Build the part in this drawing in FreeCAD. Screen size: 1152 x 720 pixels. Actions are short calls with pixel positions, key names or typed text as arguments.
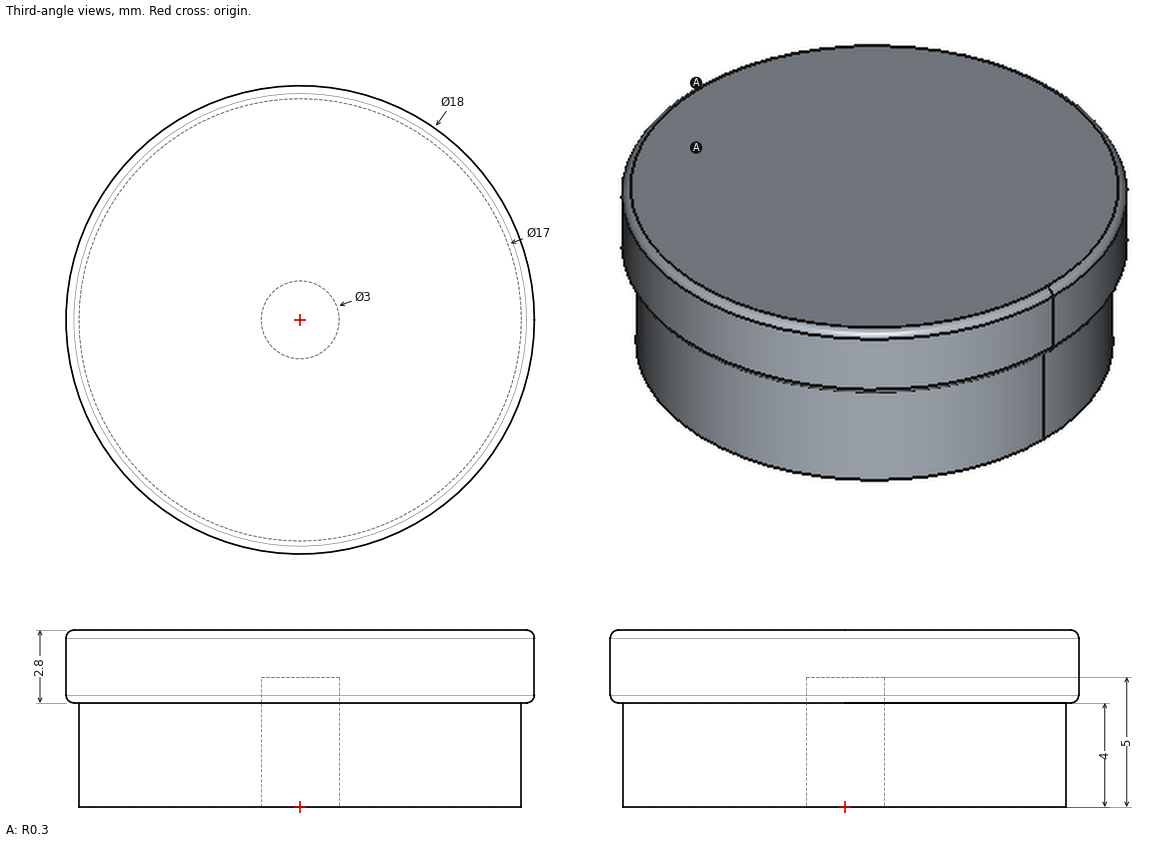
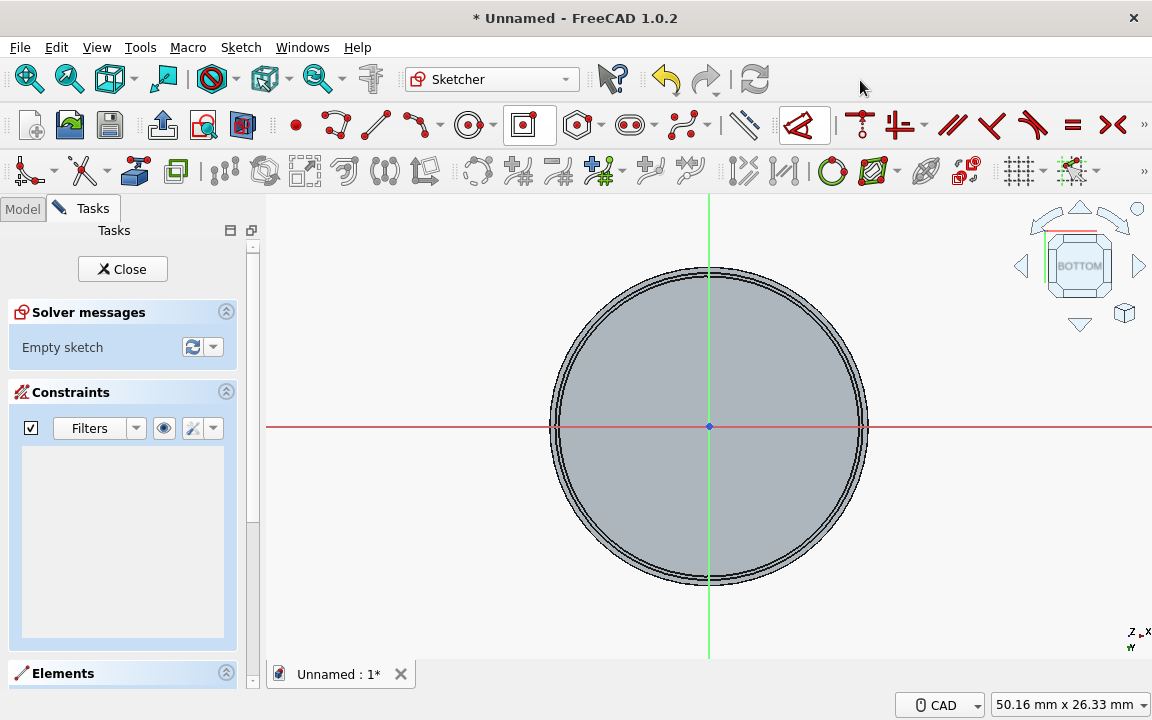
scroll(726, 426, up, 8)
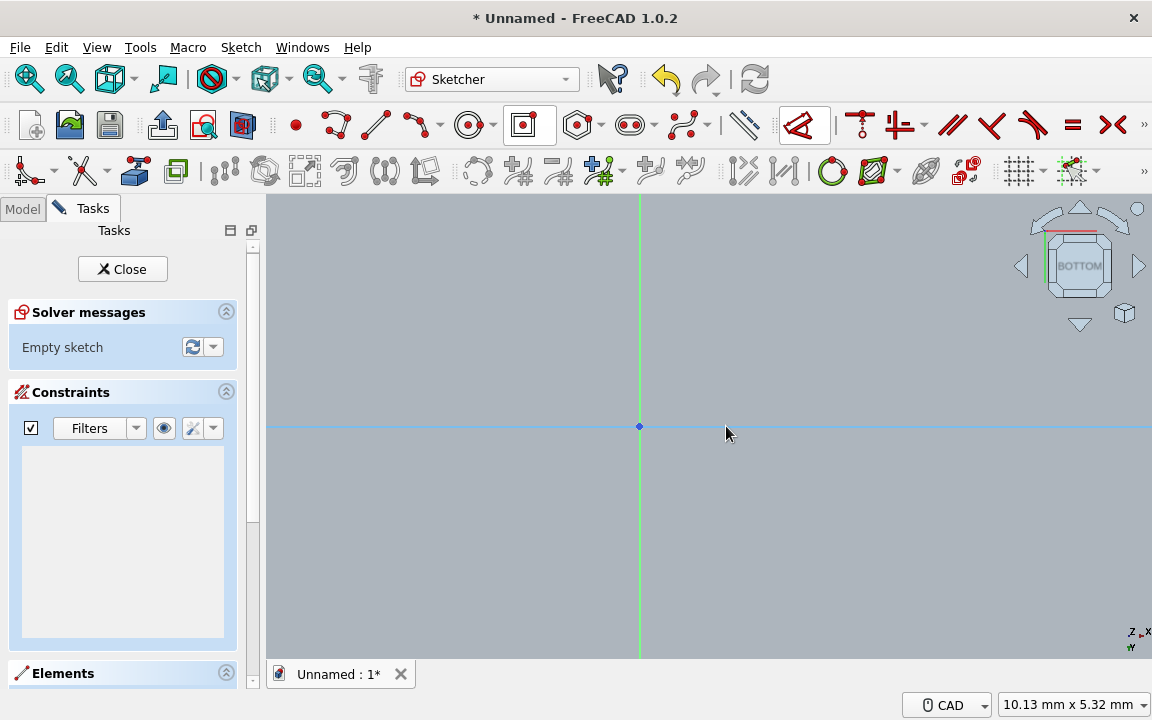
key(g)
key(c)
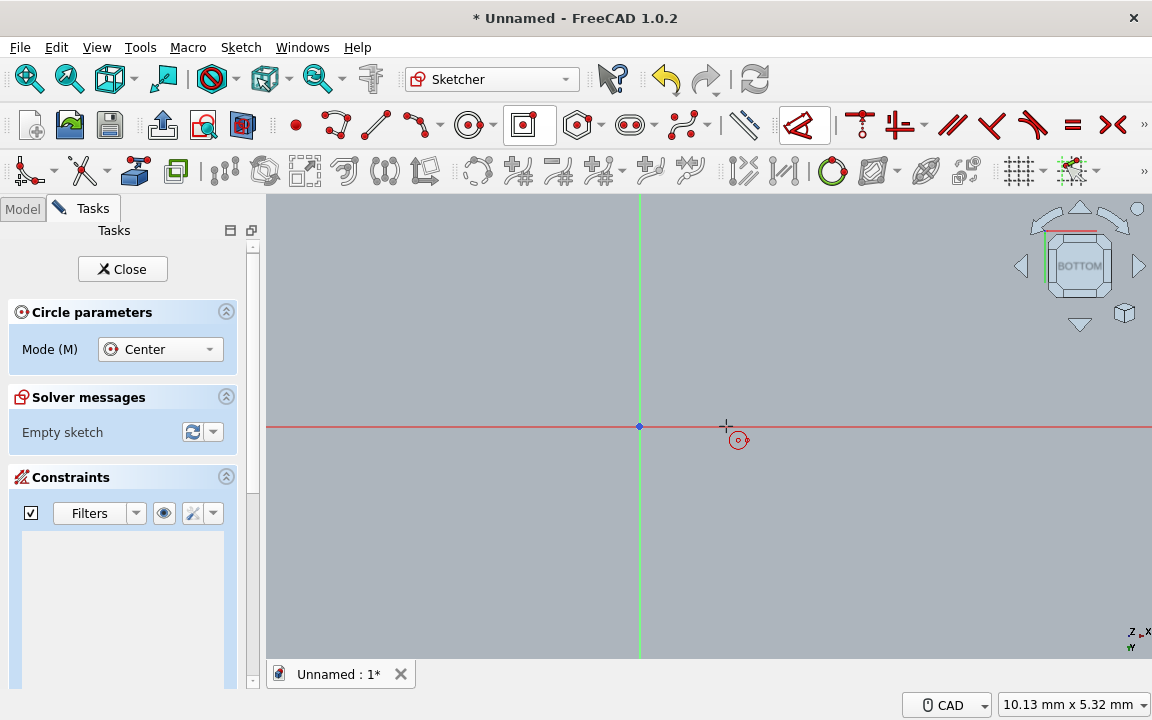
click(640, 426)
move(733, 334)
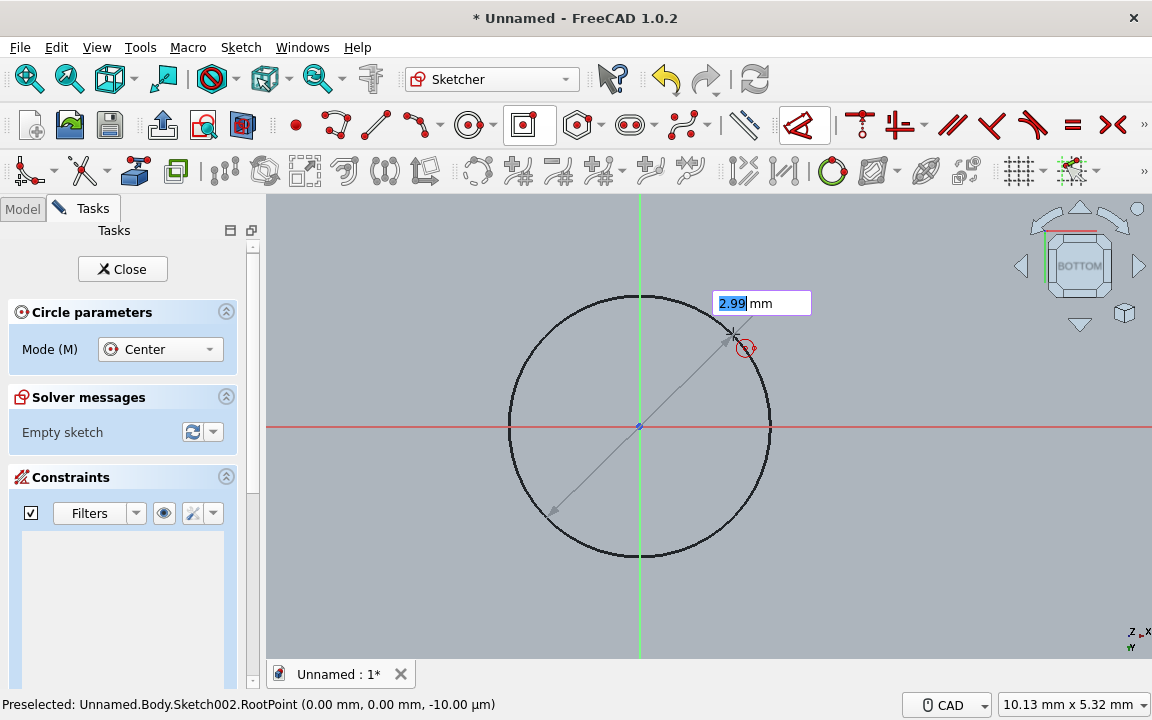
text(3)
key(Return)
key(Escape)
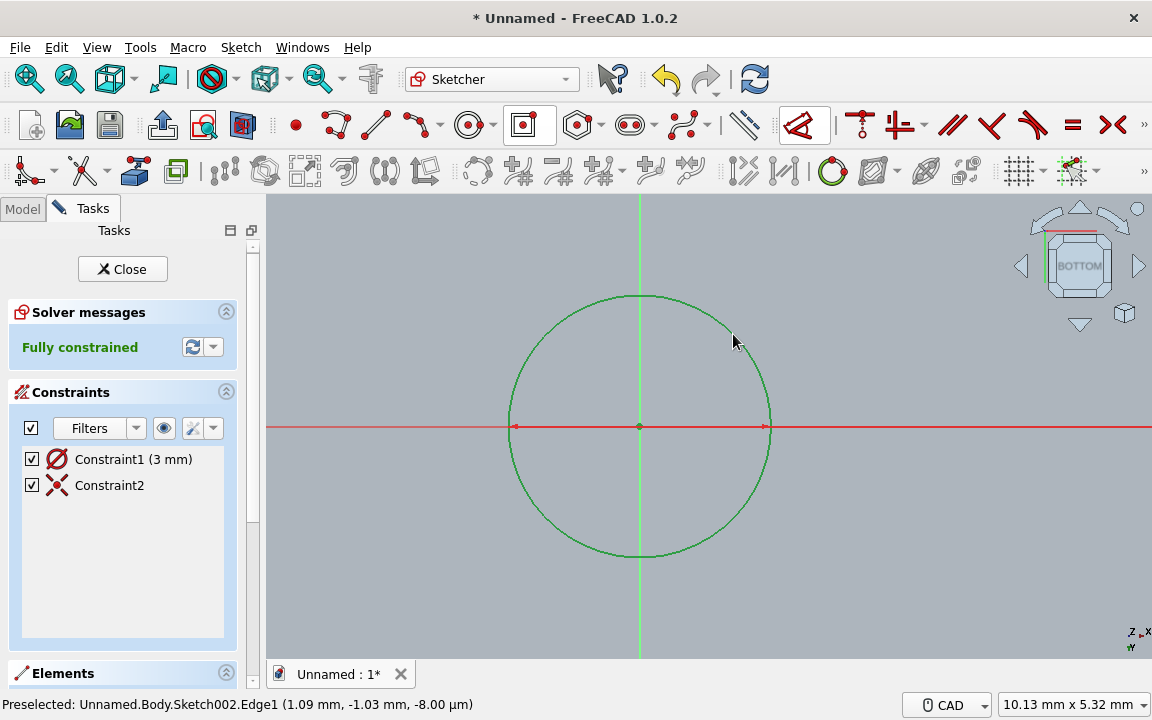
click(123, 269)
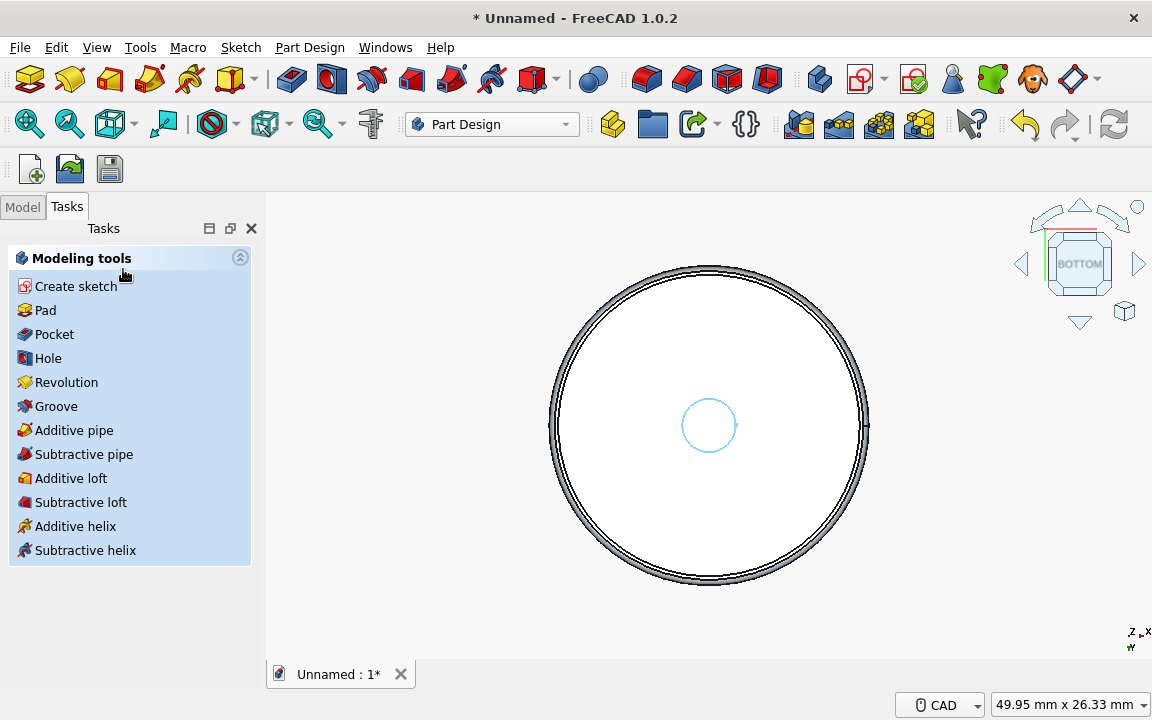
click(292, 80)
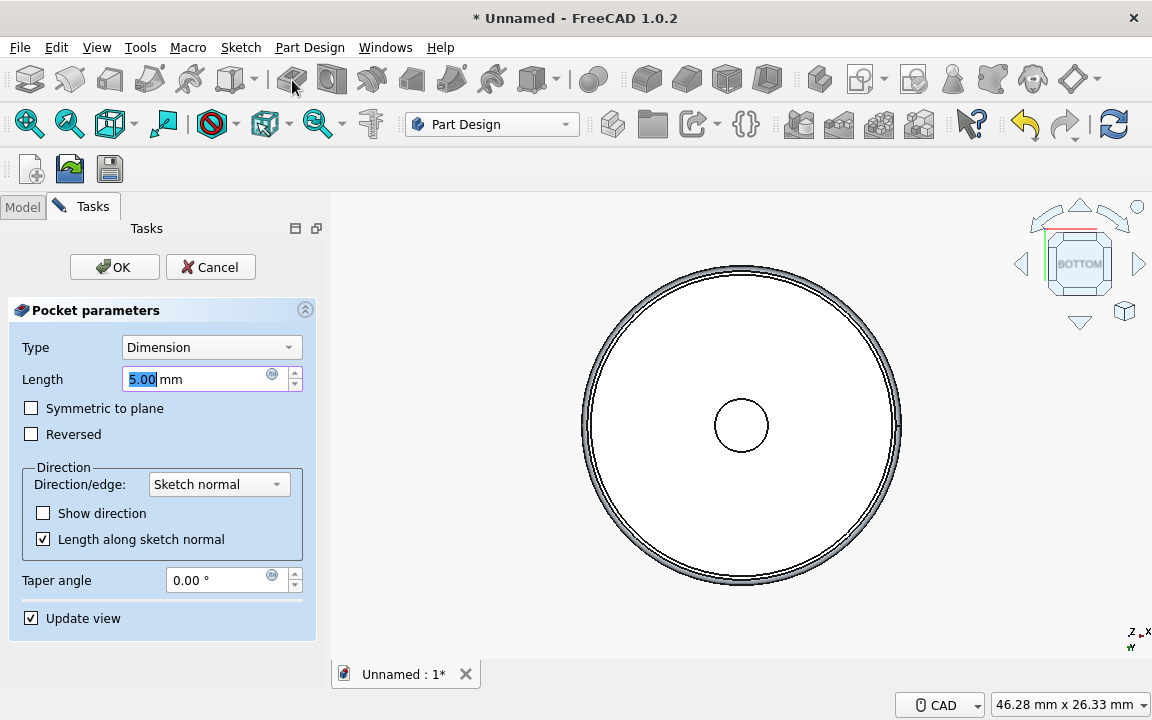
text(5)
key(Tab)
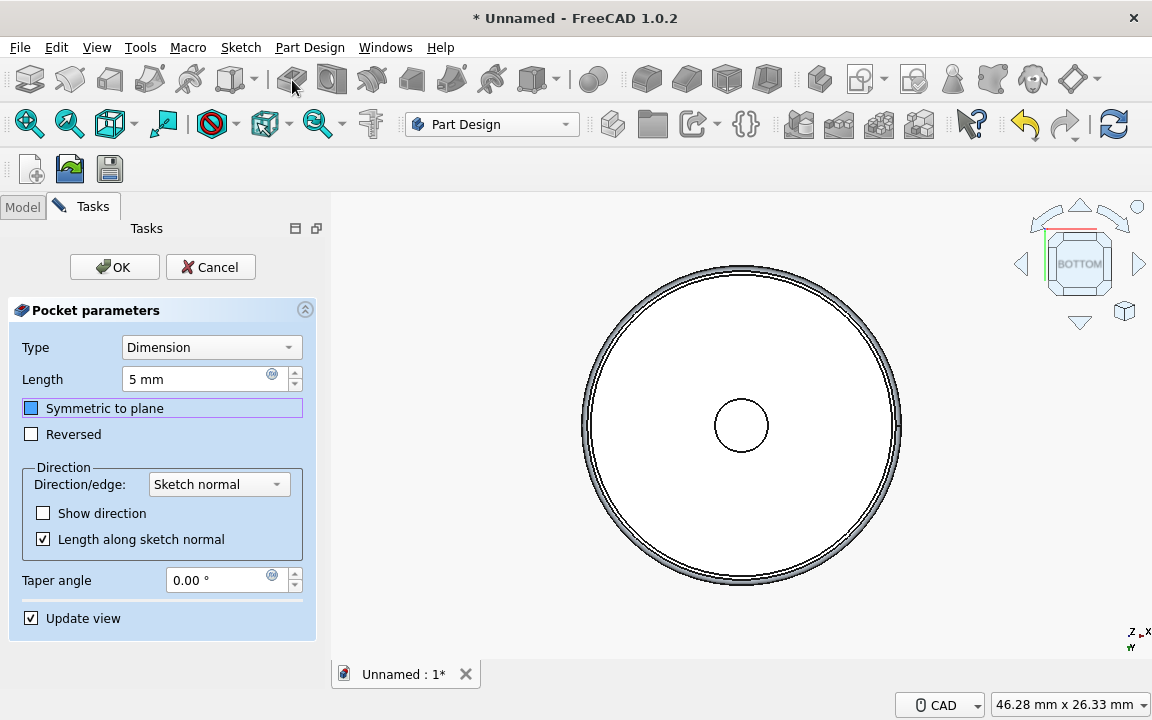
click(115, 267)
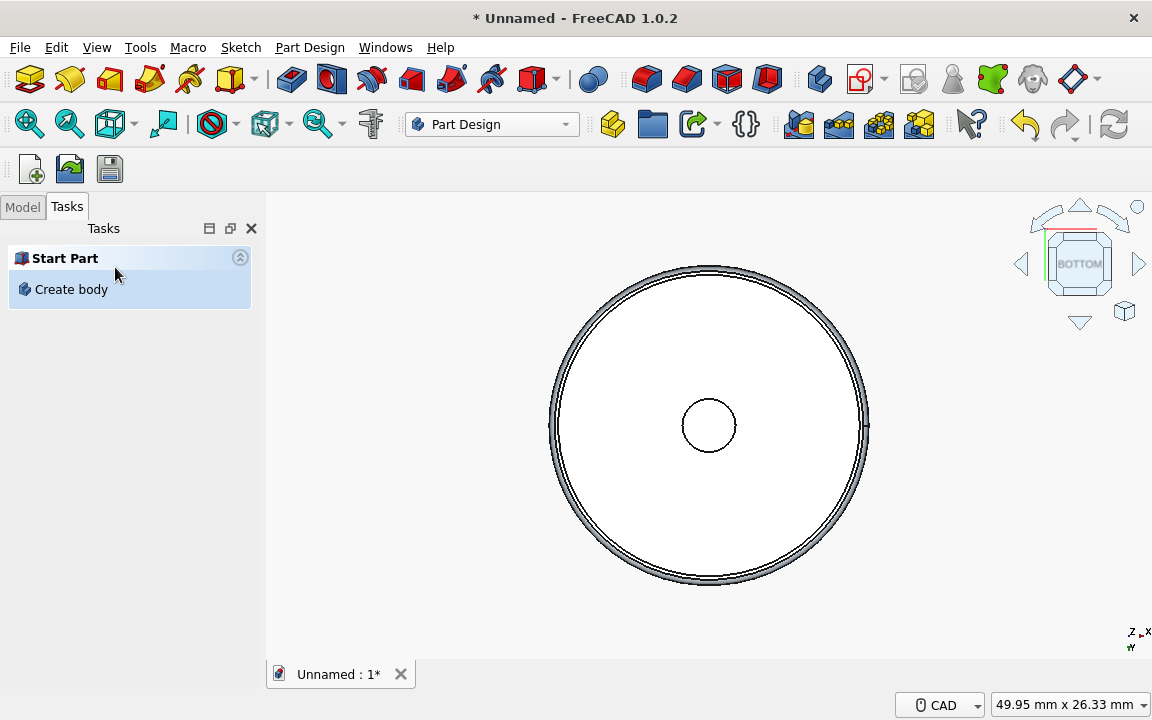
key(0)